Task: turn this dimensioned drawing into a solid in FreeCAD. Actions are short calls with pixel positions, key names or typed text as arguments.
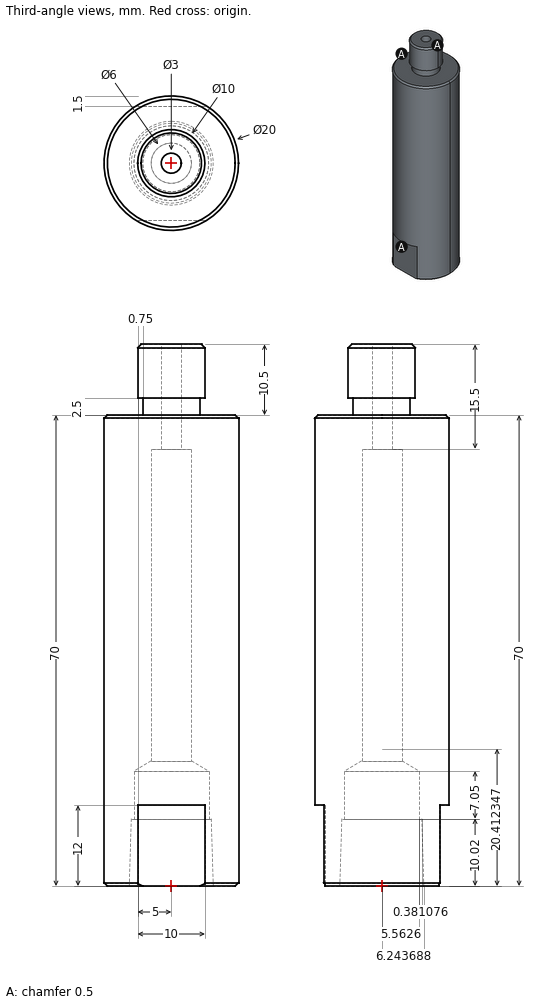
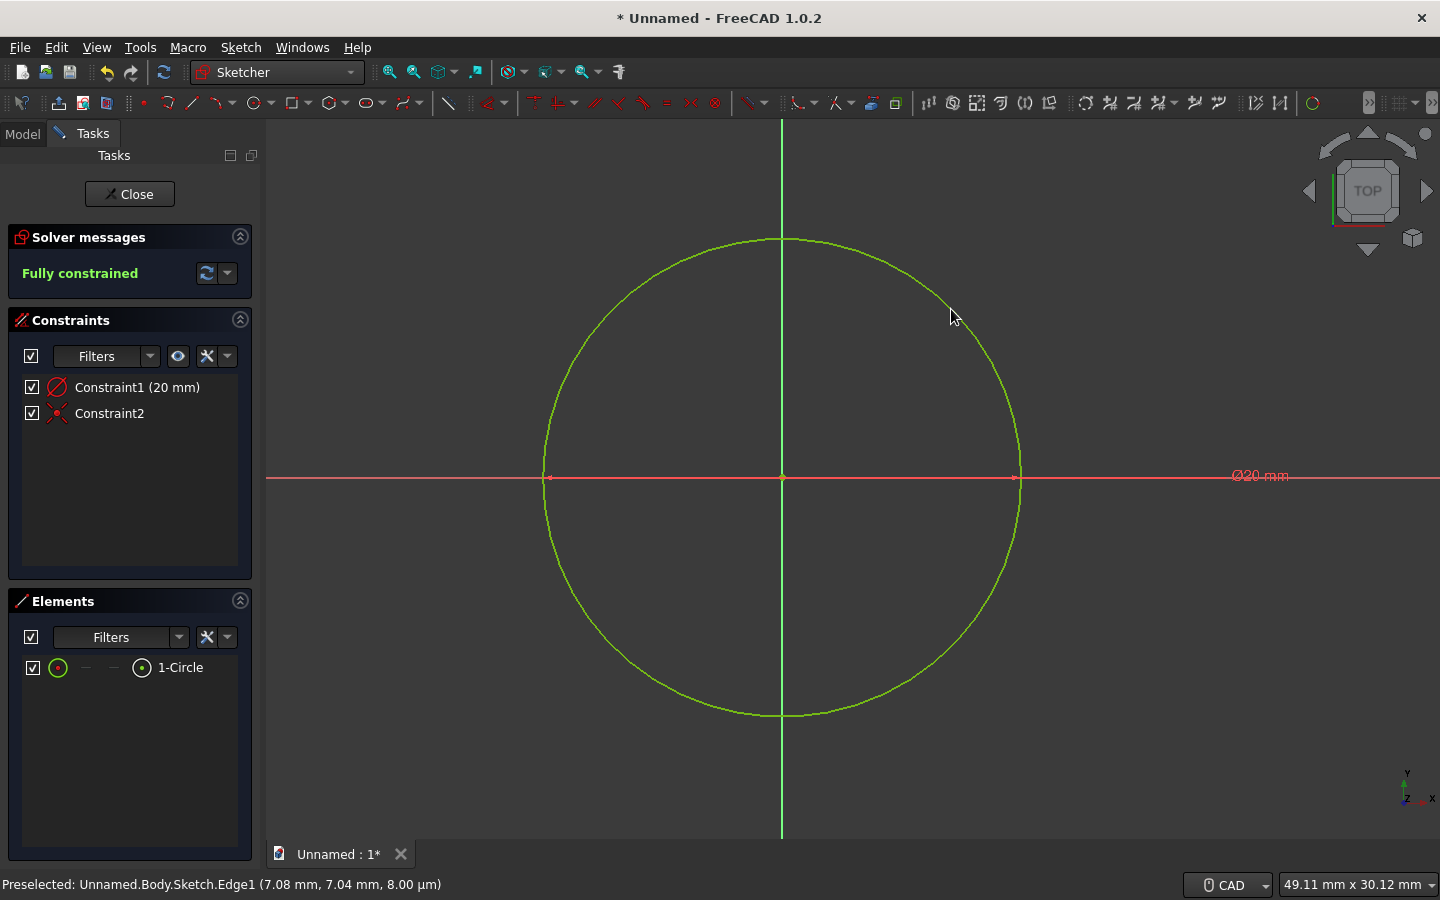
click(130, 194)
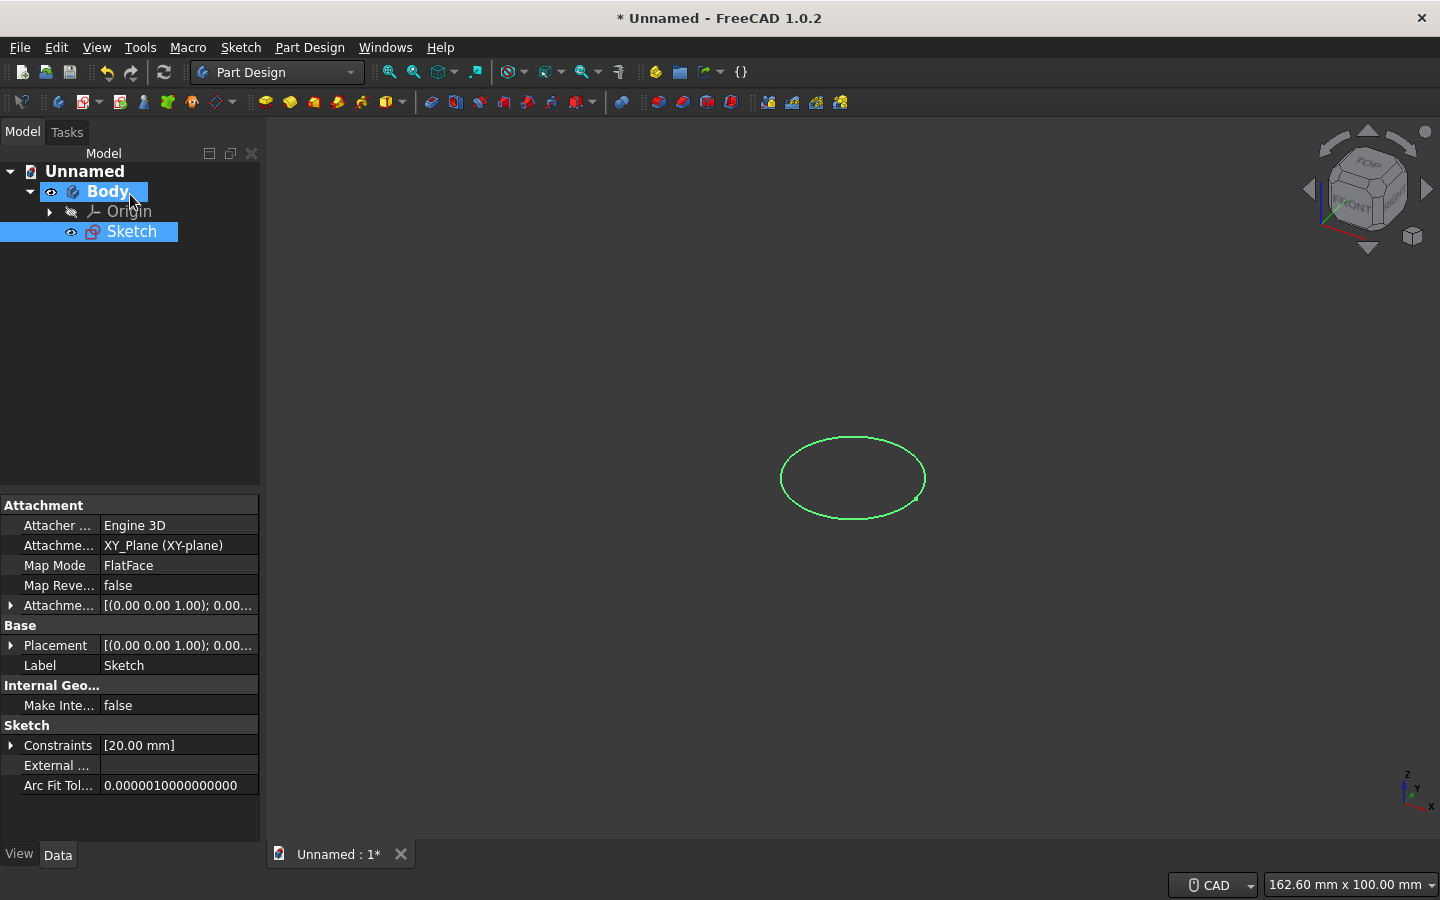
click(266, 102)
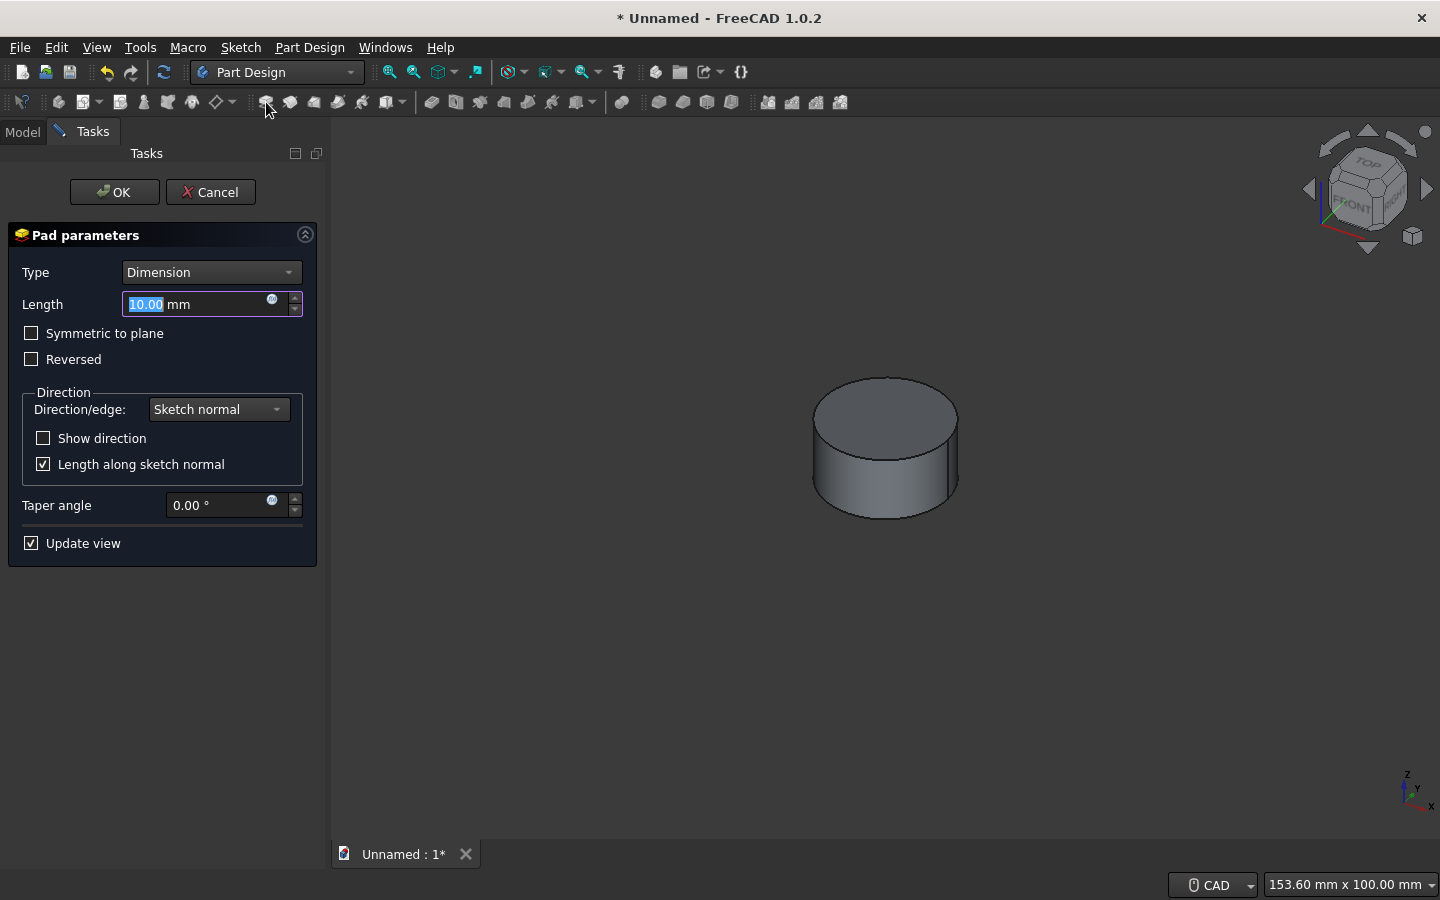
text(70)
key(Tab)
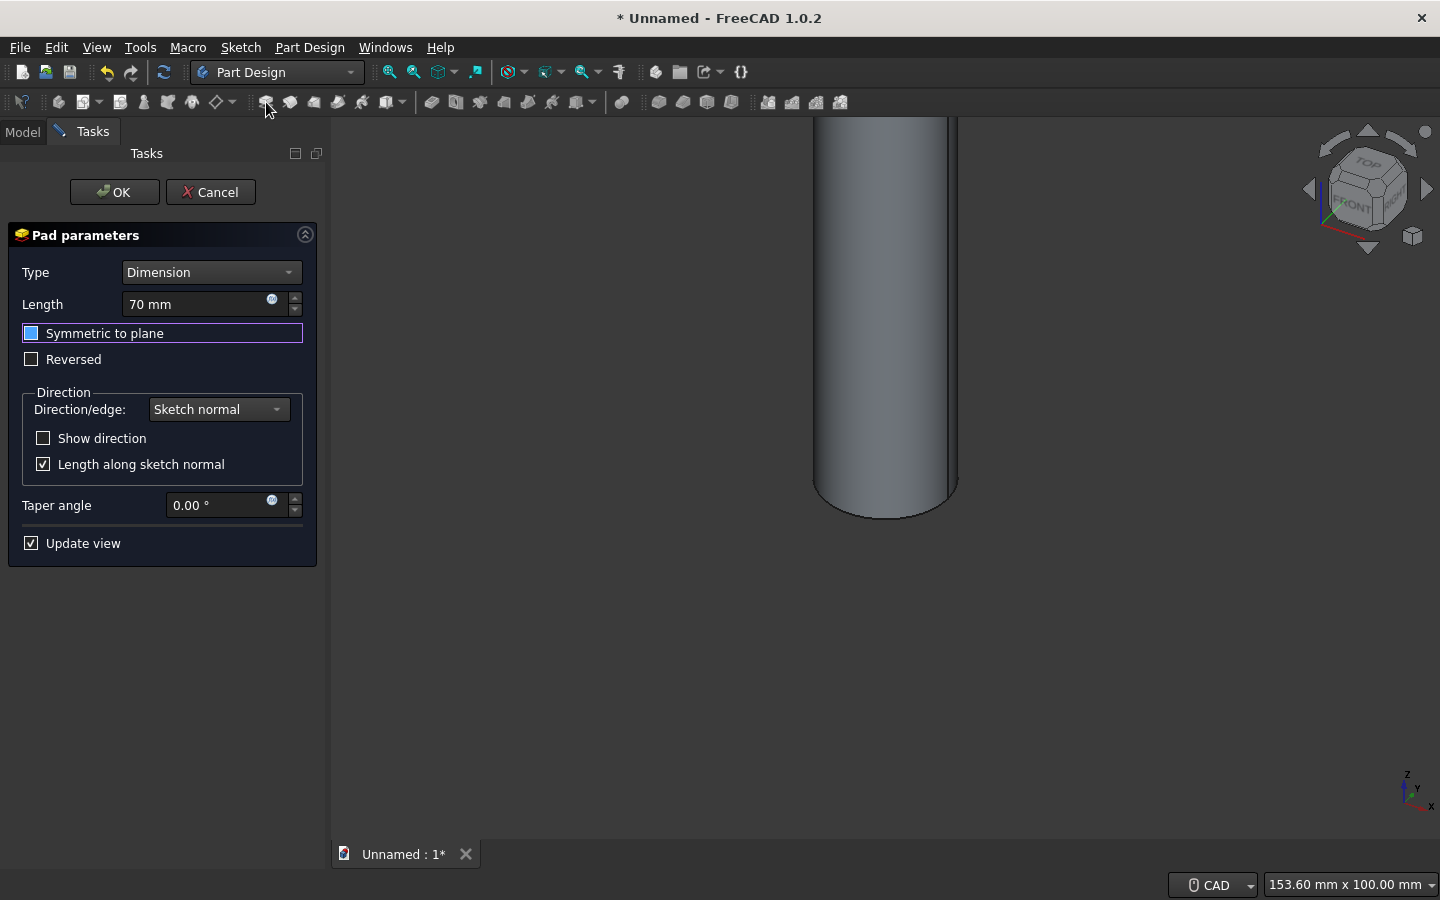
click(115, 192)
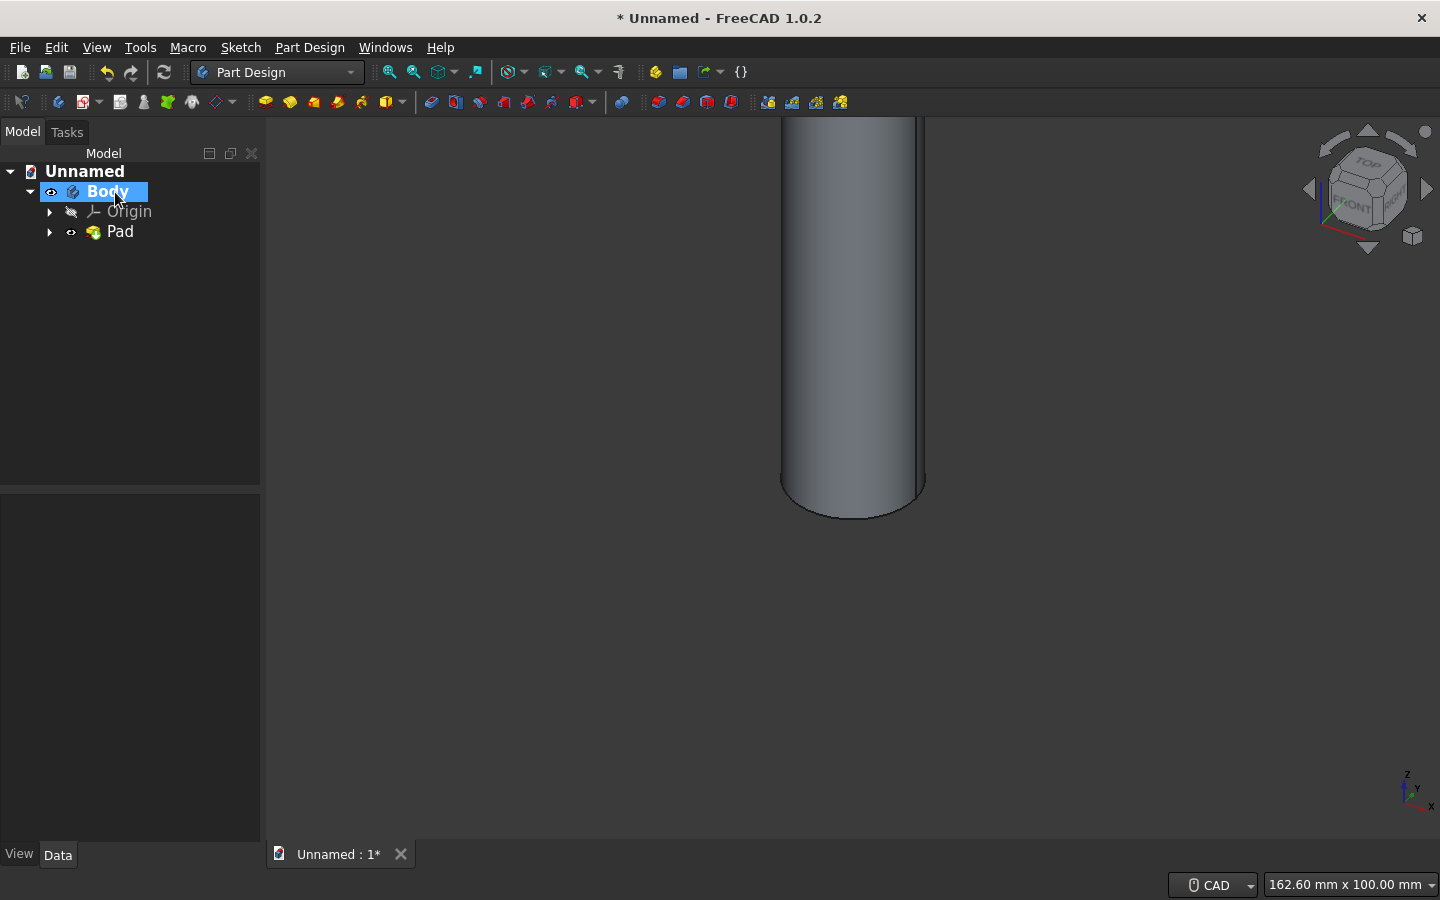
key(v)
key(f)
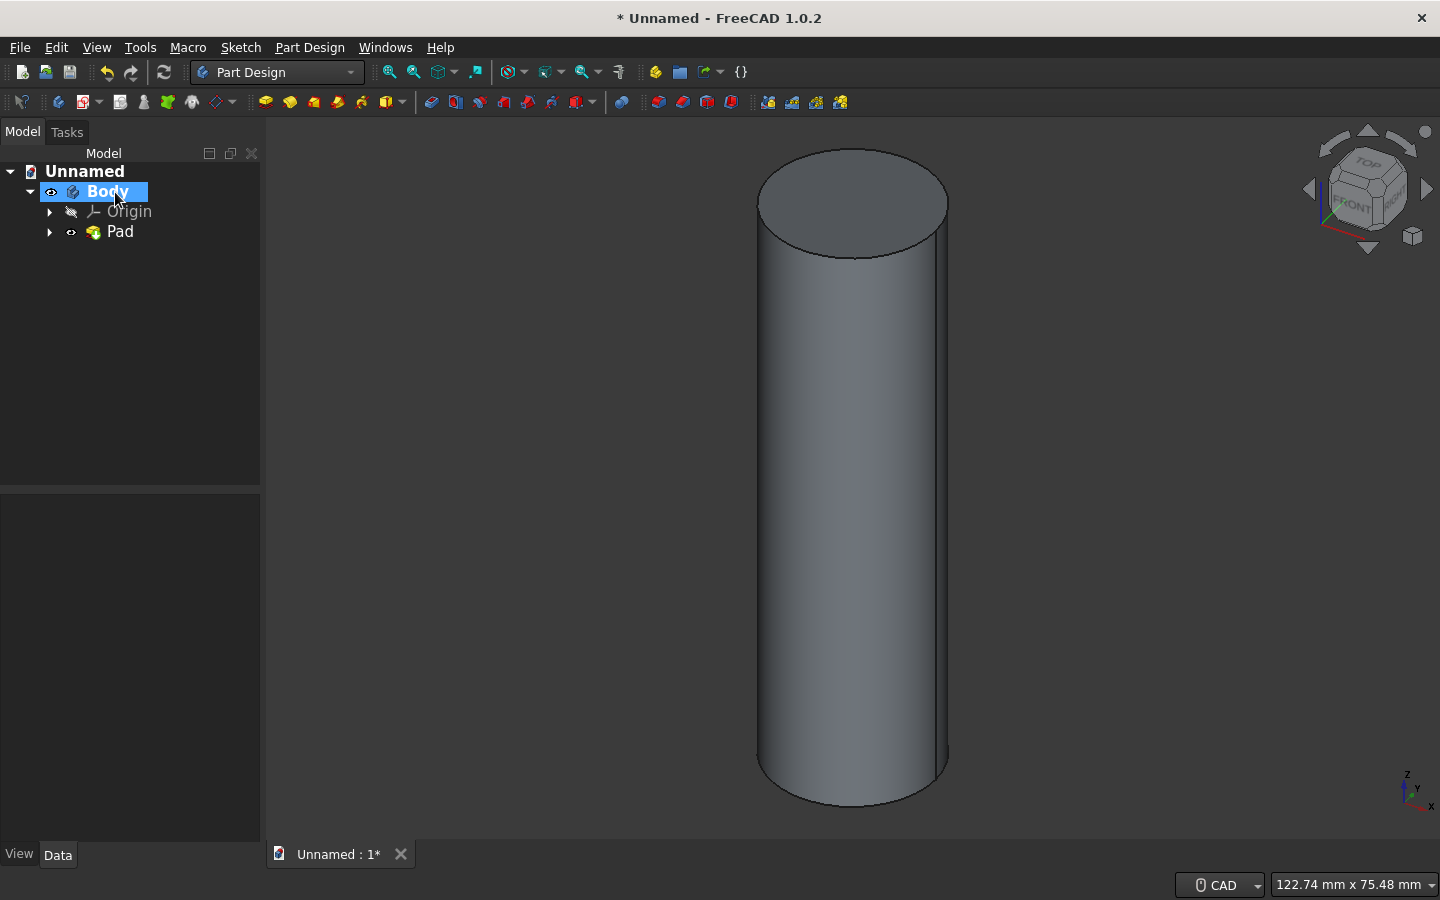
click(853, 203)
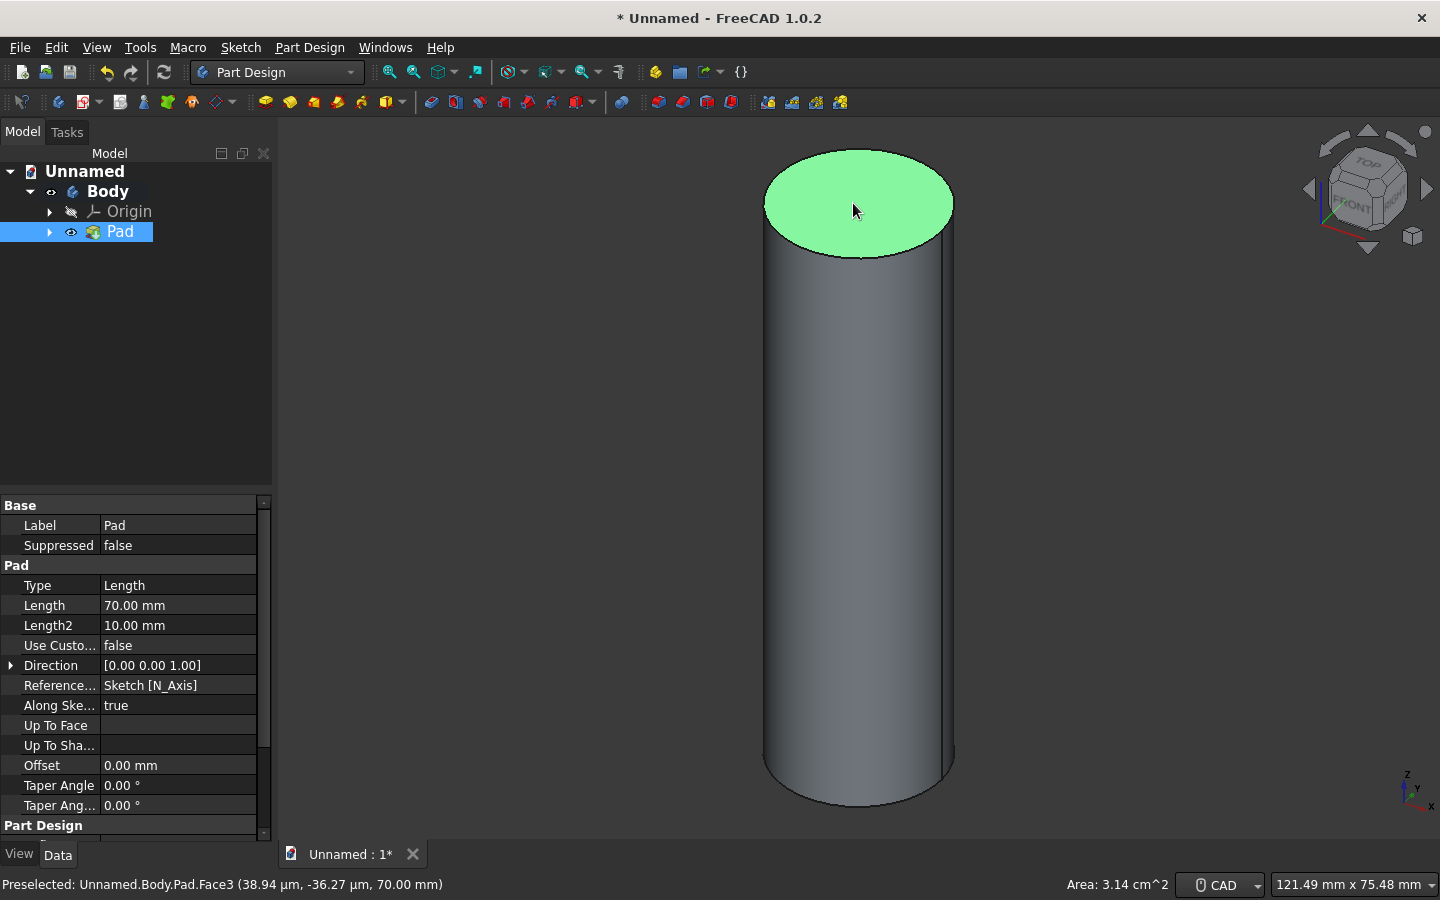
click(84, 102)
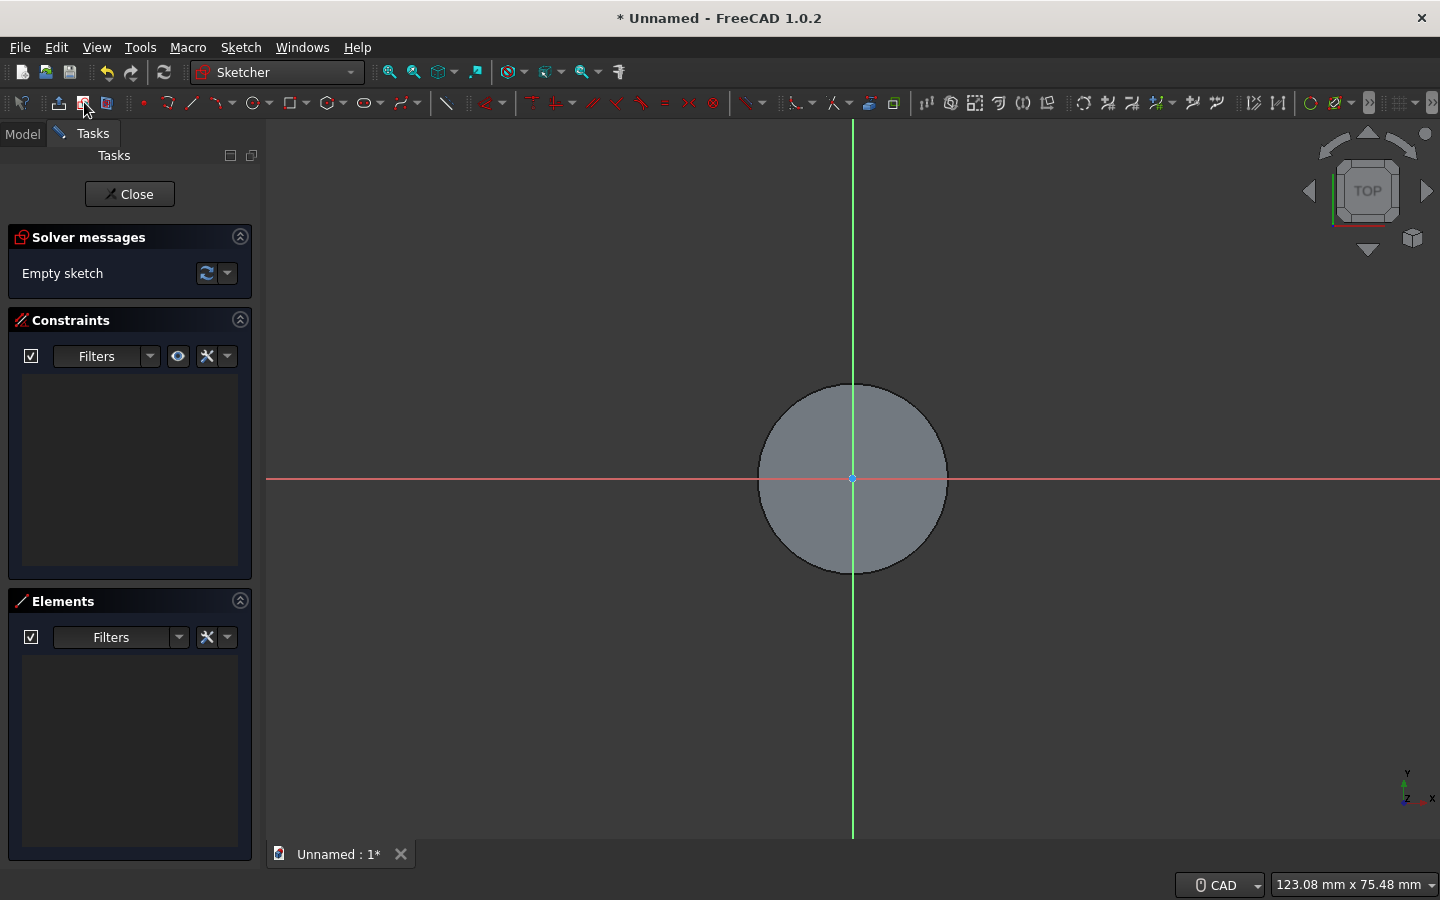
scroll(870, 479, up, 8)